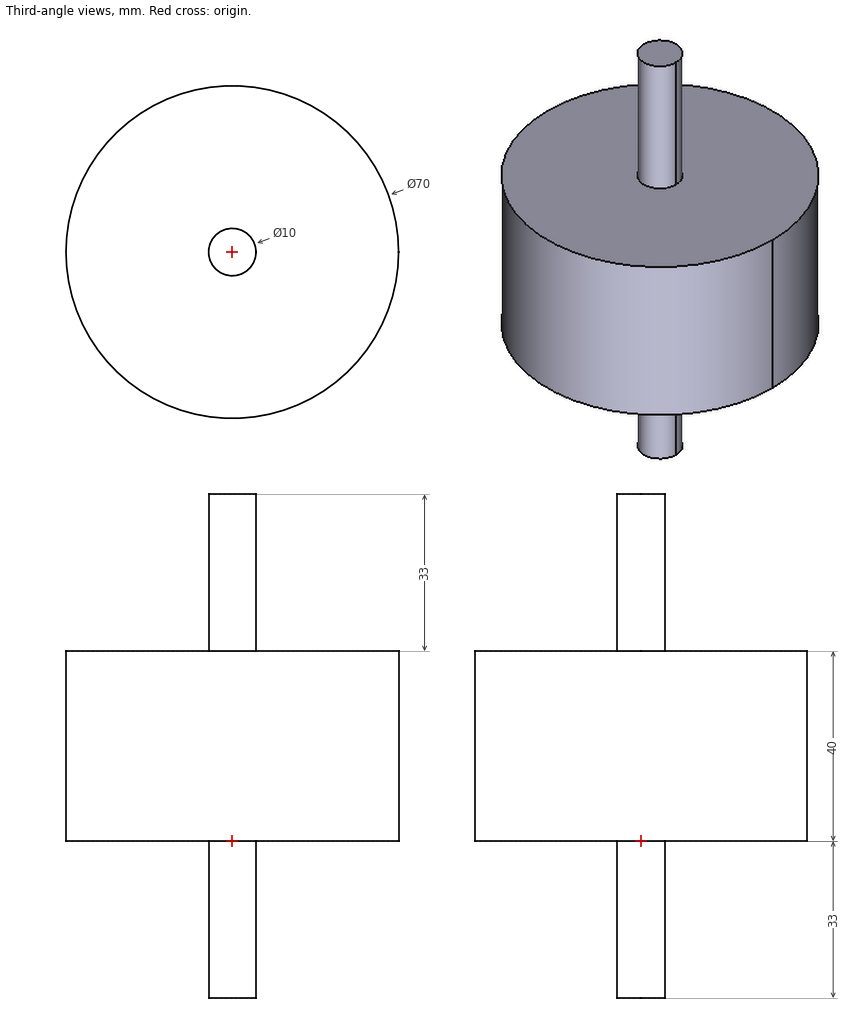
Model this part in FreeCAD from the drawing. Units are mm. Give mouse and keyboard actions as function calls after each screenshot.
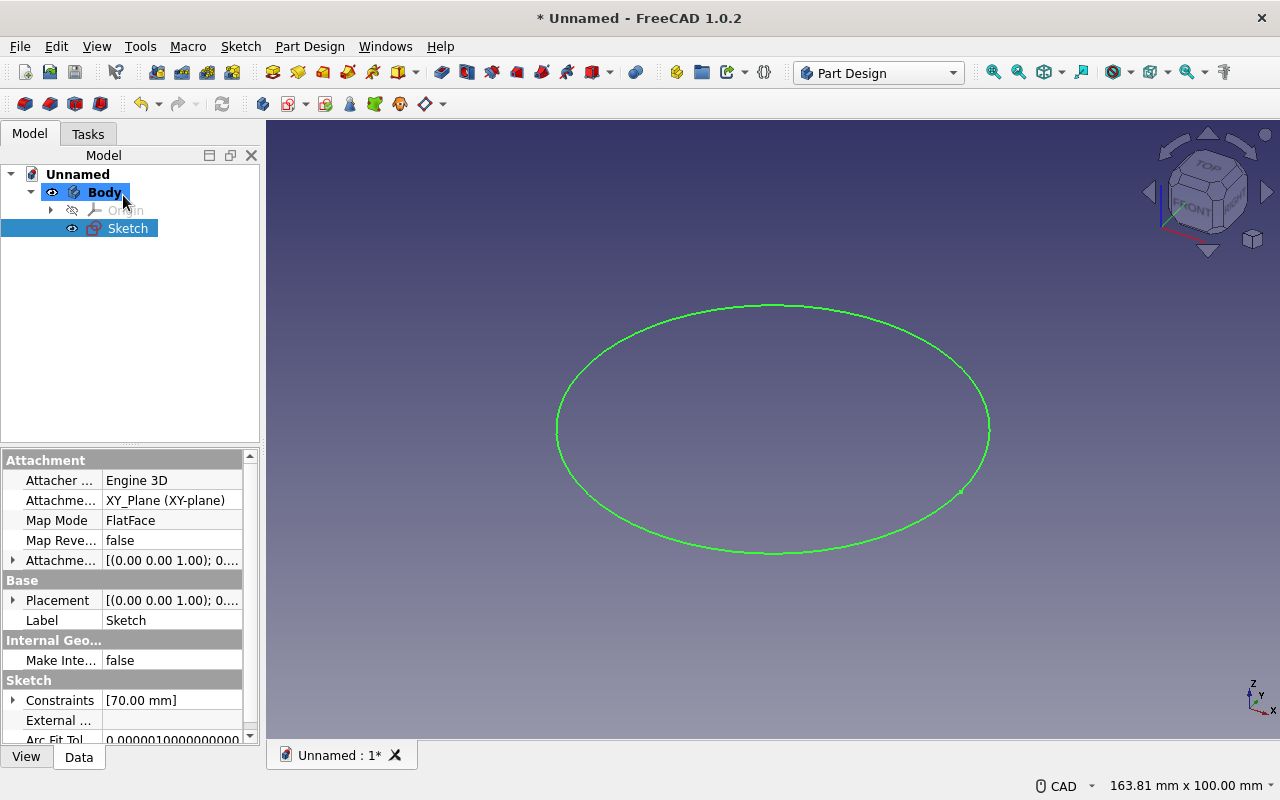
click(273, 72)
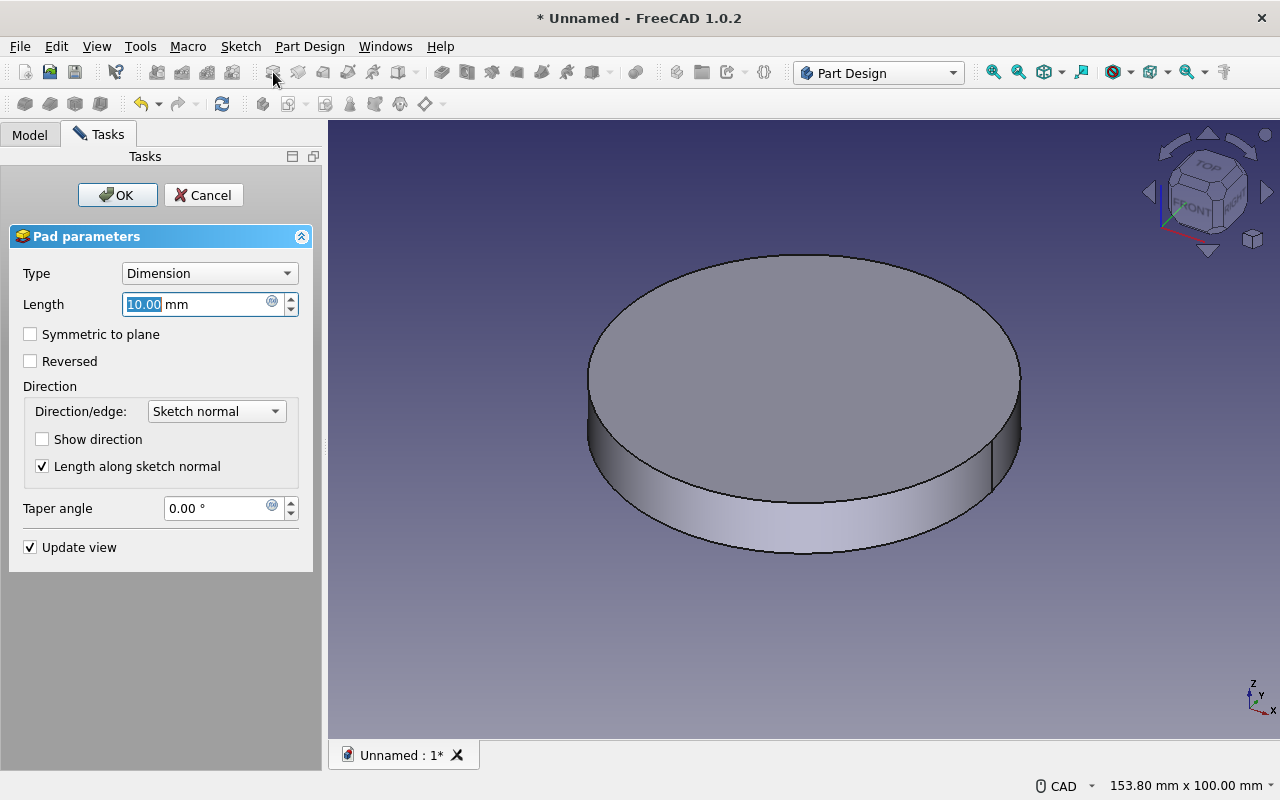
text(40)
key(Tab)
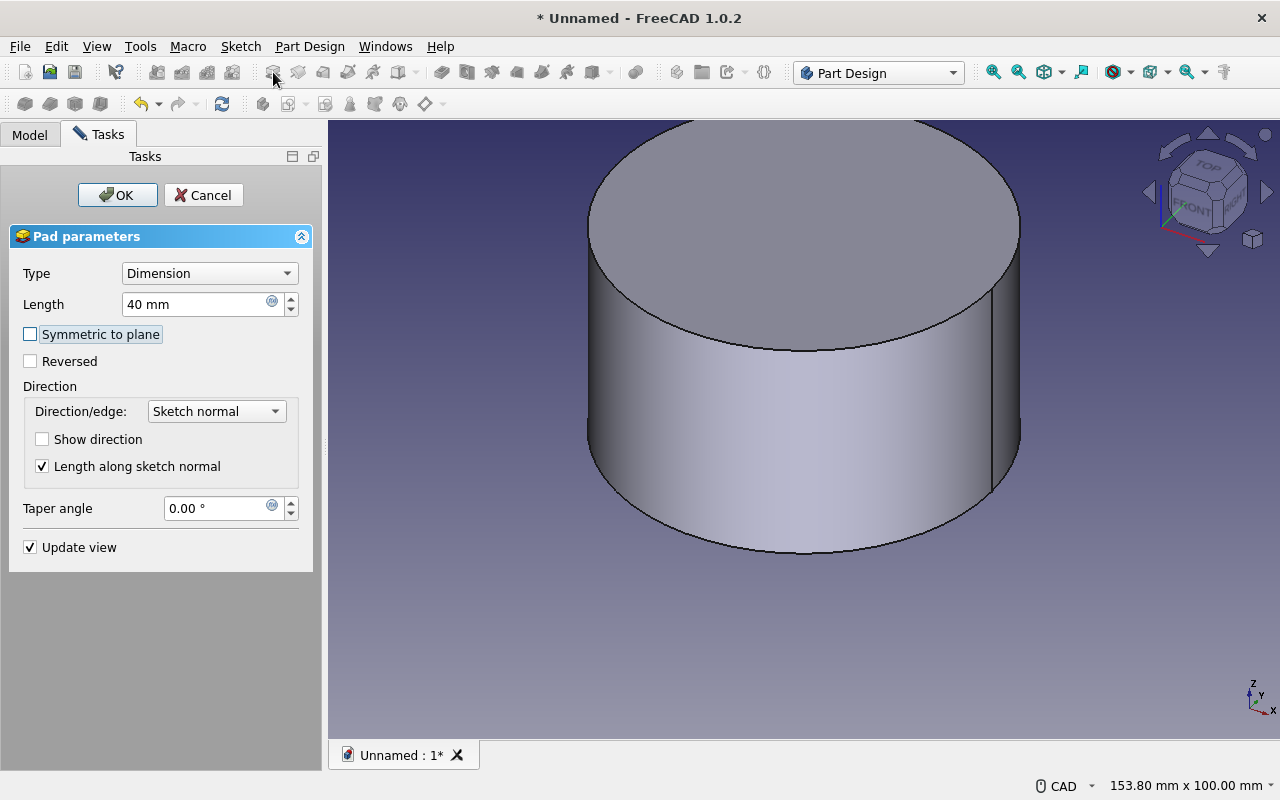
click(118, 195)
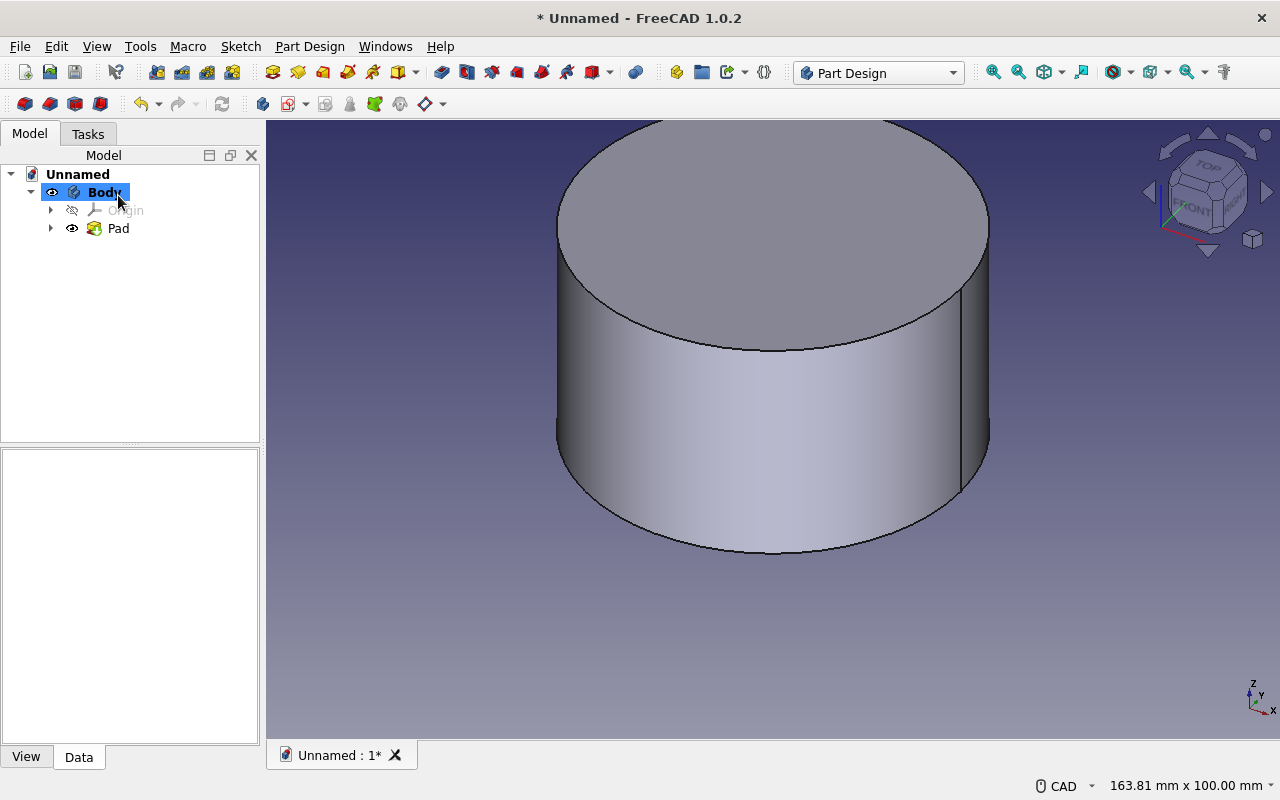
key(v)
key(f)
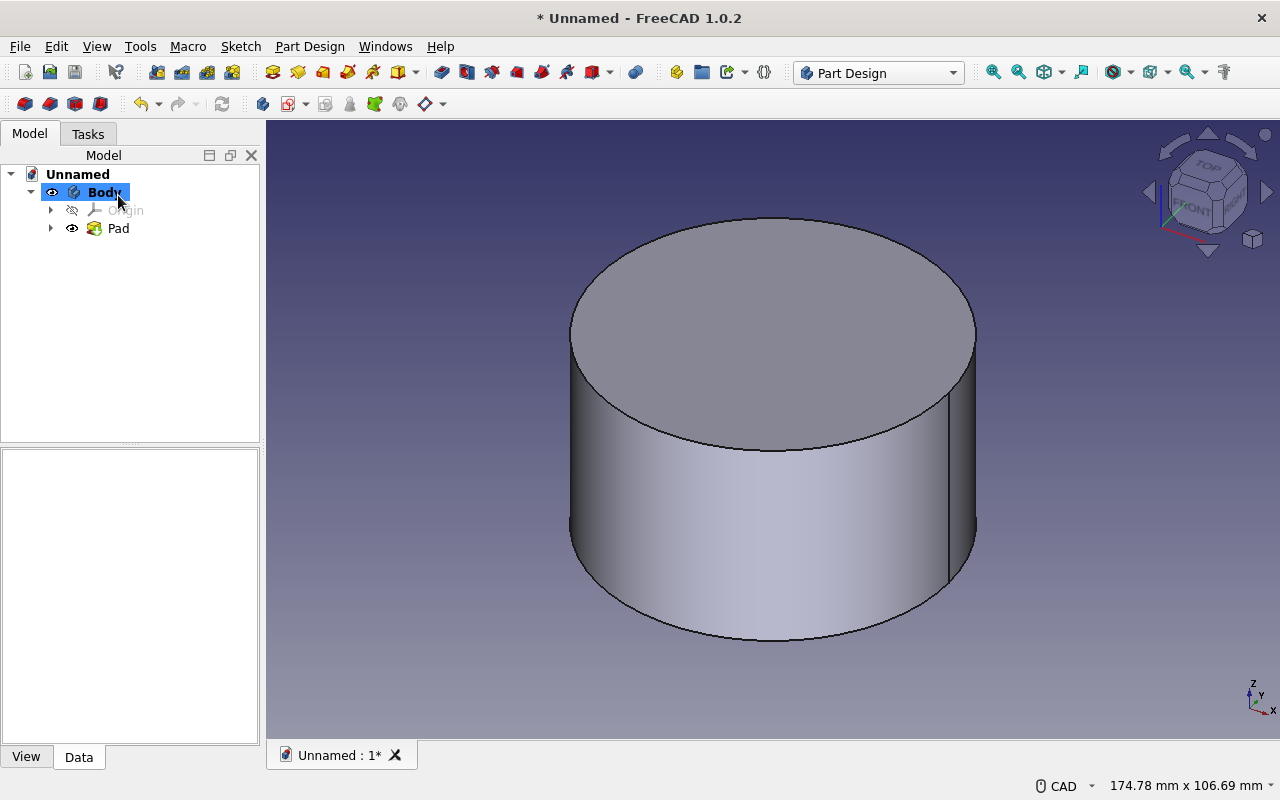
click(773, 333)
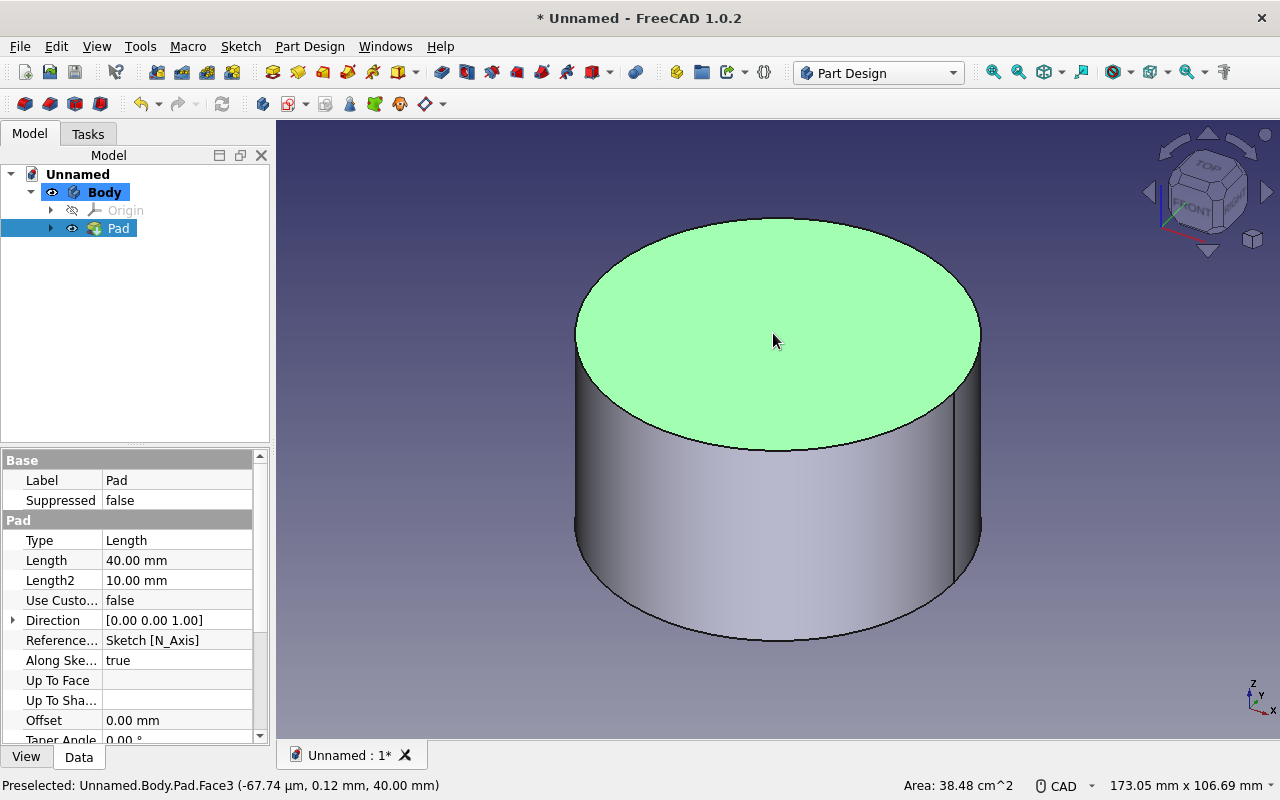
click(288, 104)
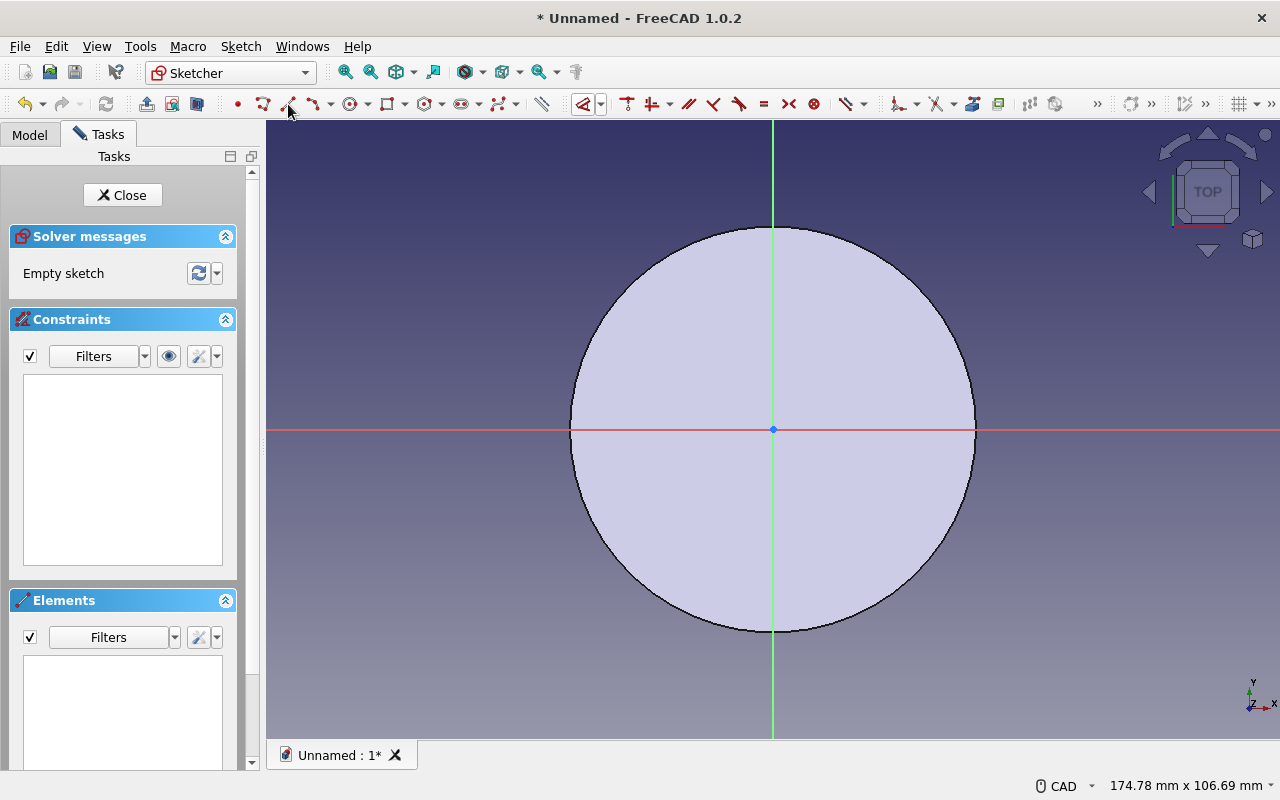
scroll(784, 430, up, 10)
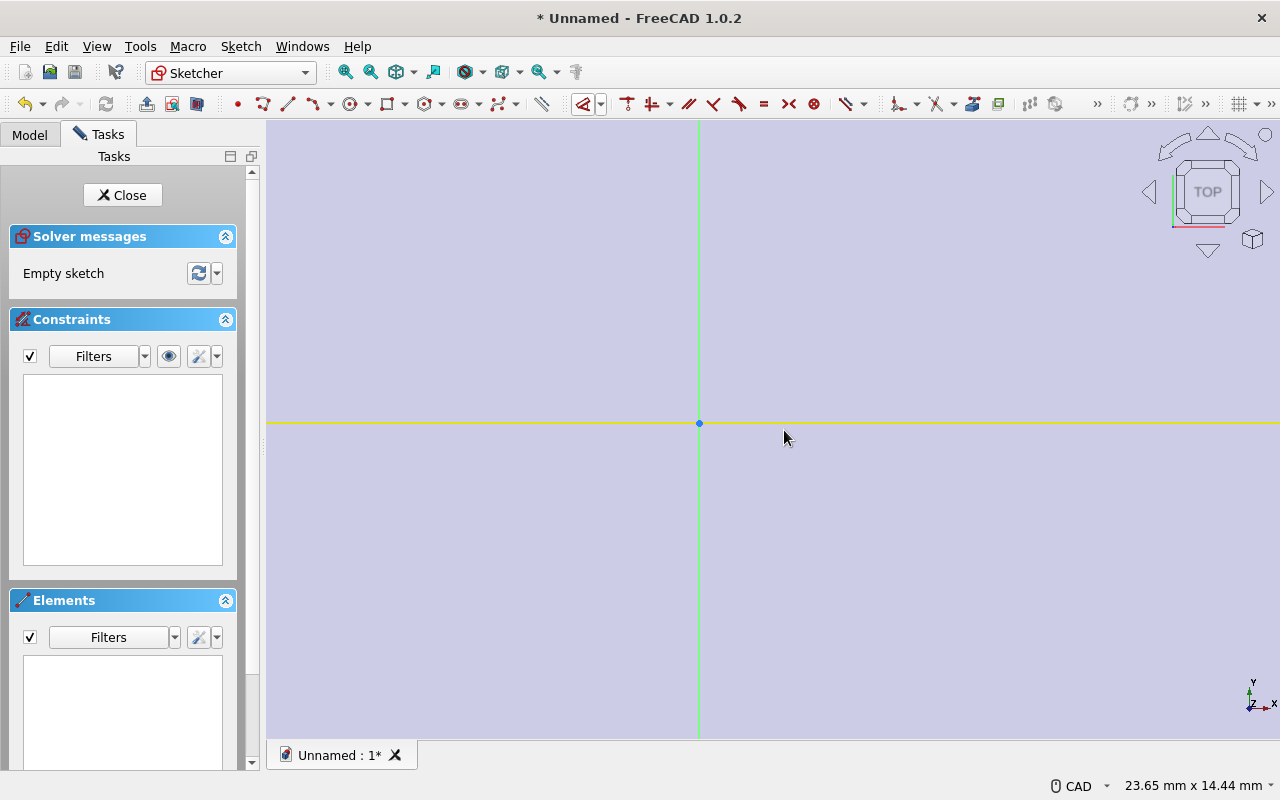
key(g)
key(c)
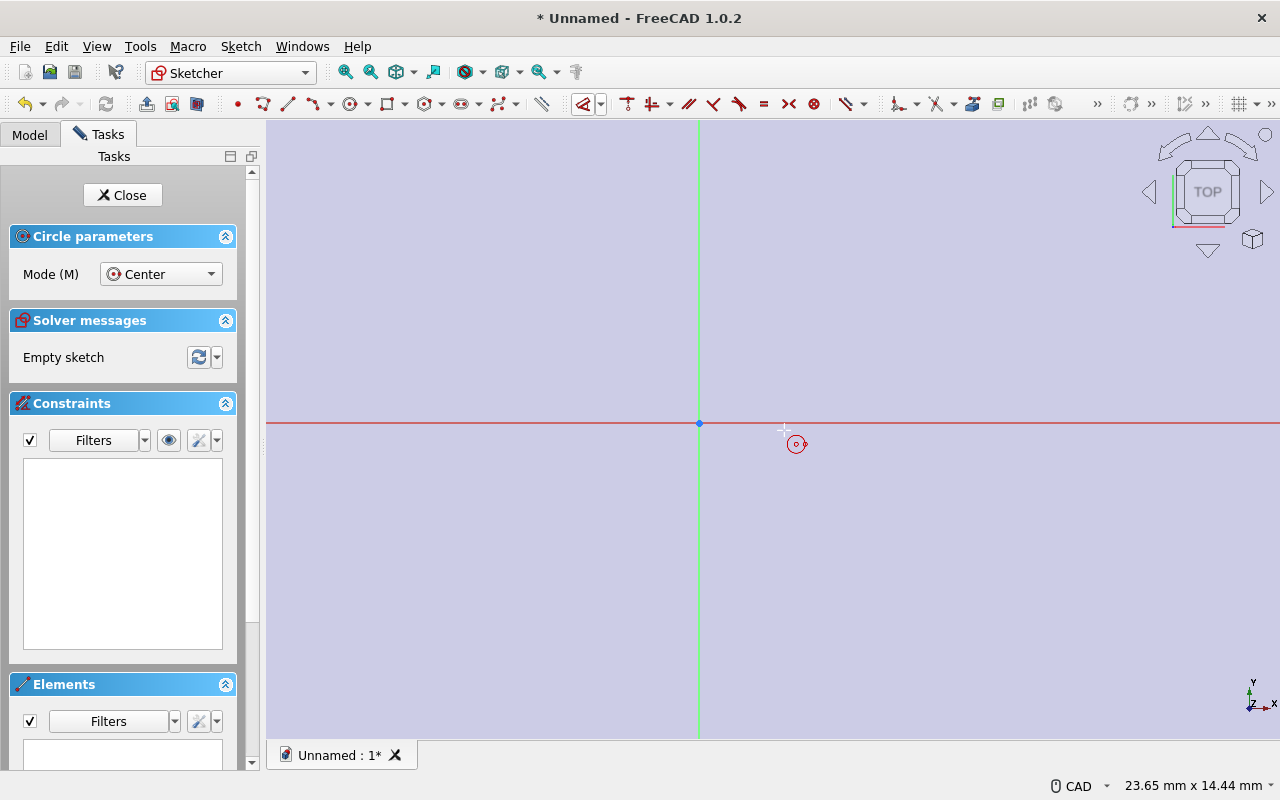
click(699, 423)
click(851, 272)
key(Escape)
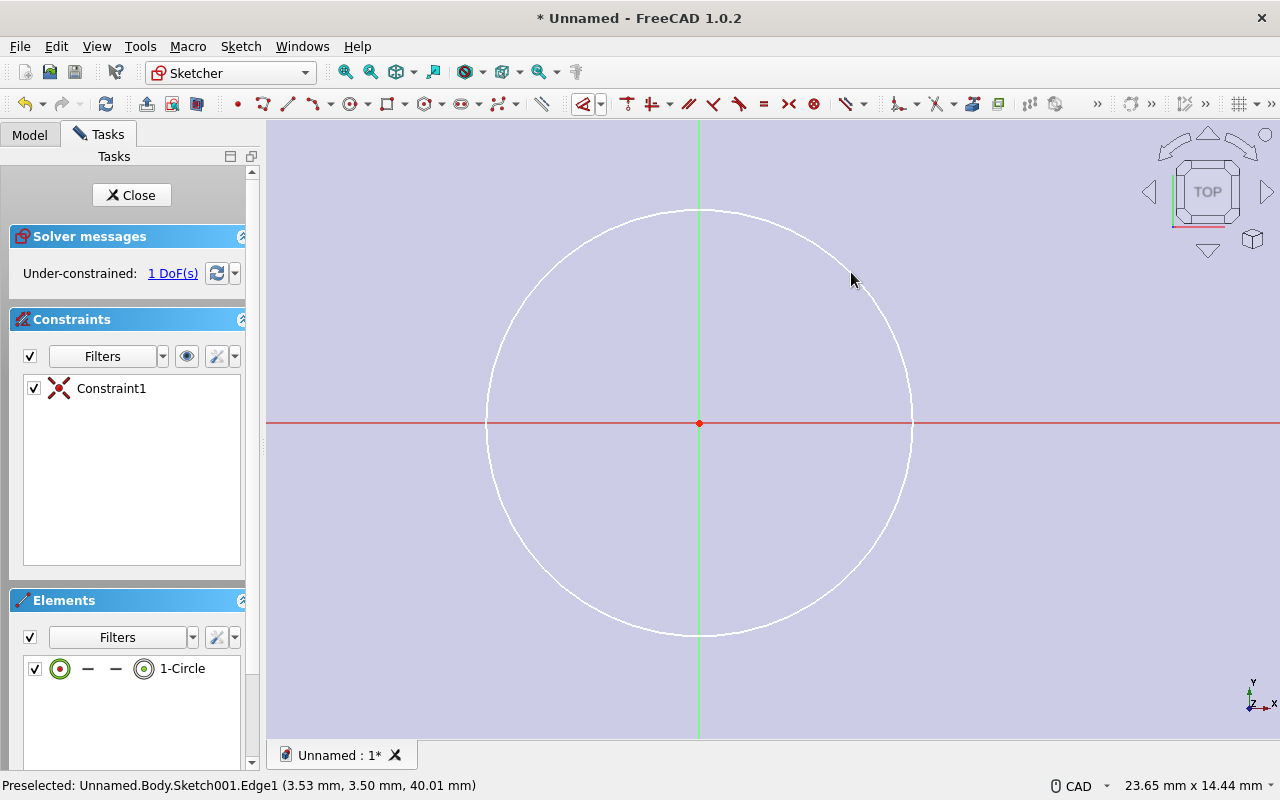
key(d)